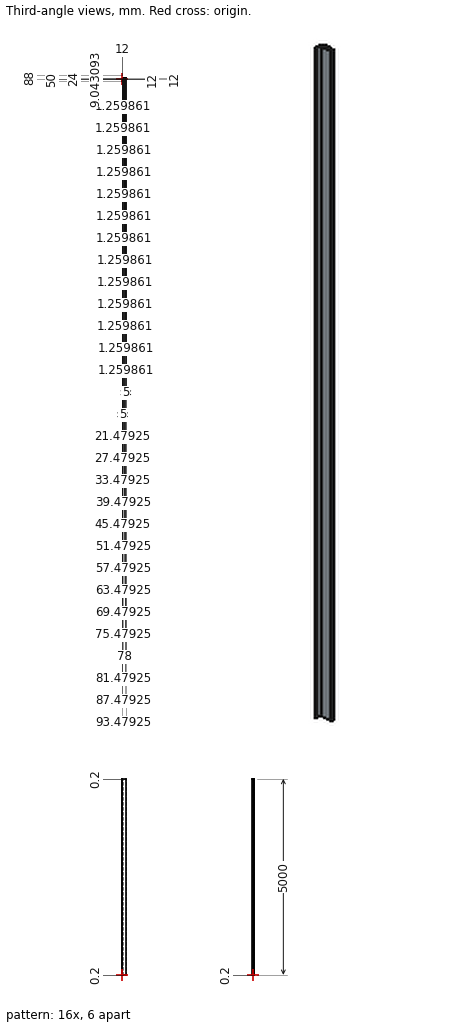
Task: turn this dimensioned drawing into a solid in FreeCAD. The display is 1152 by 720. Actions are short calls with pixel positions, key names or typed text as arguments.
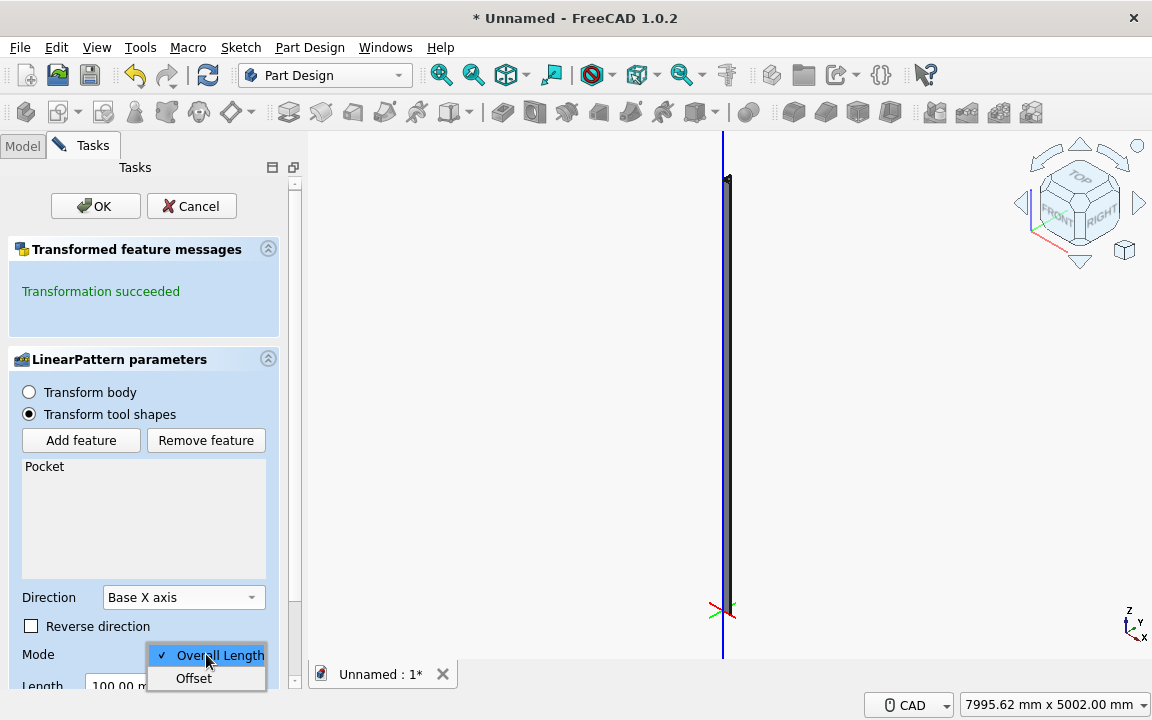
click(206, 678)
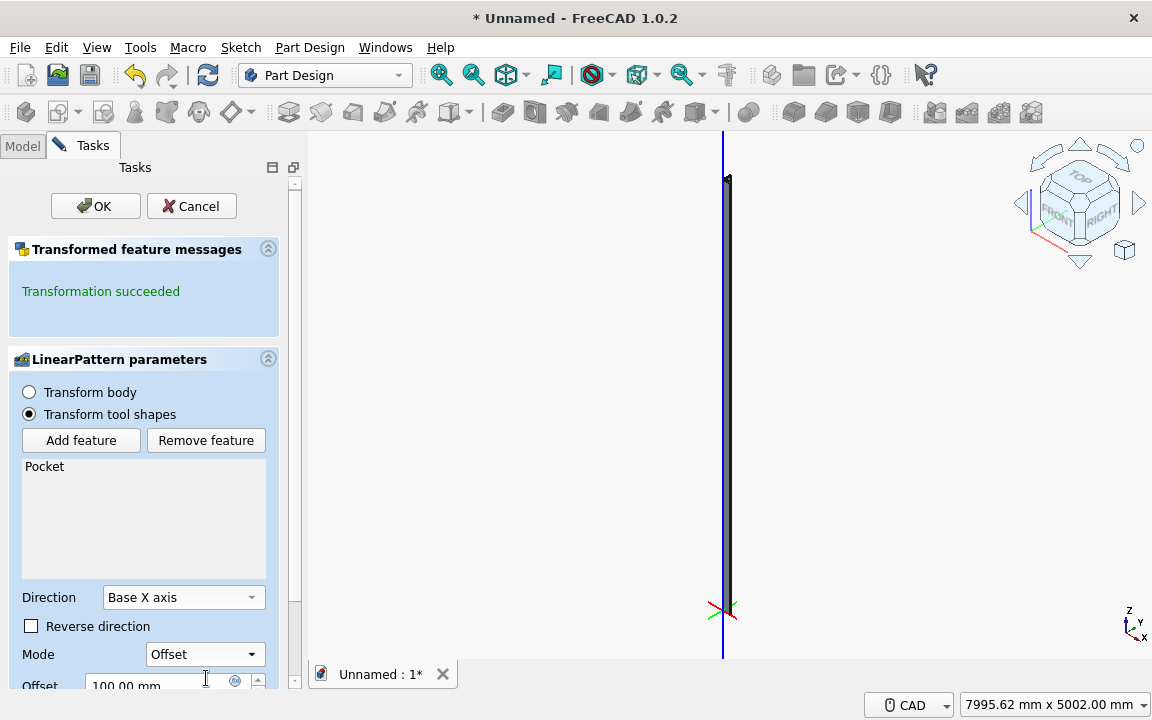
scroll(295, 432, down, 2)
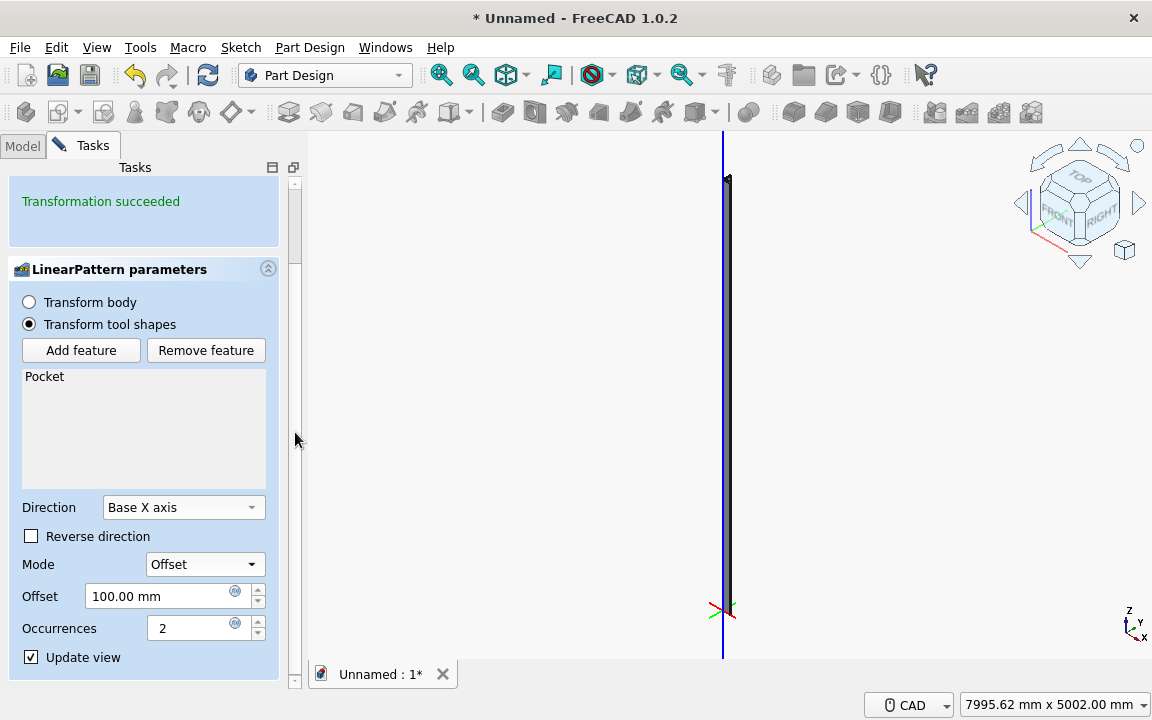
triple_click(168, 596)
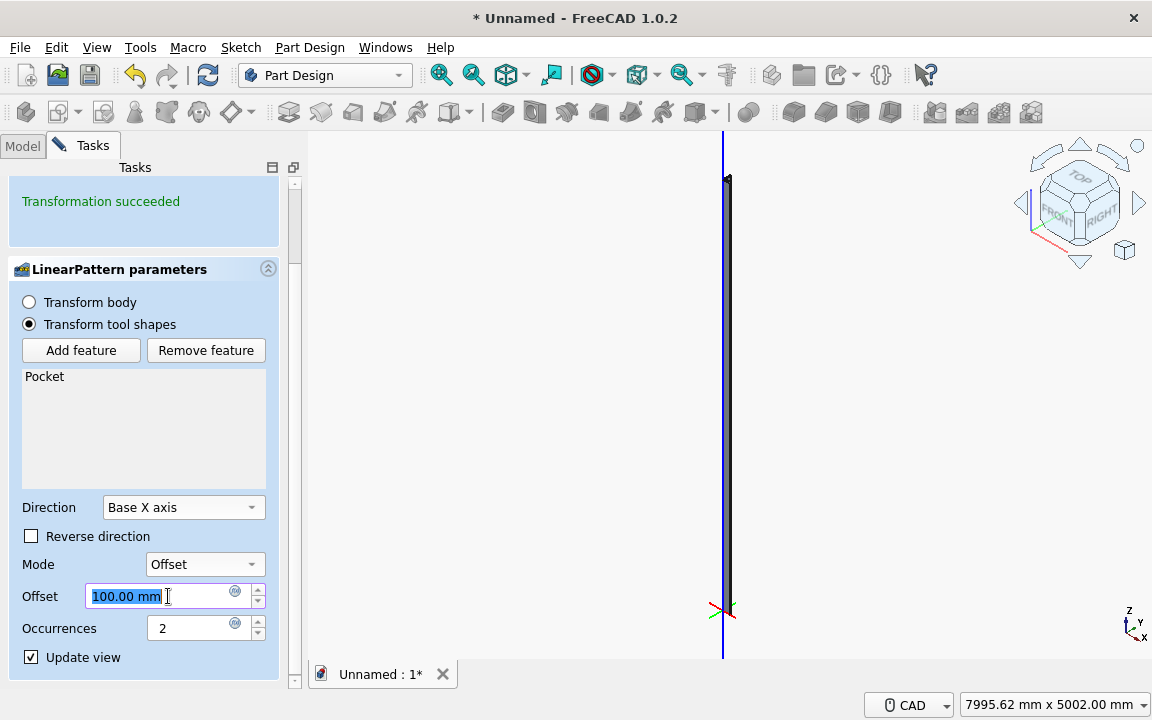
text(6)
key(Tab)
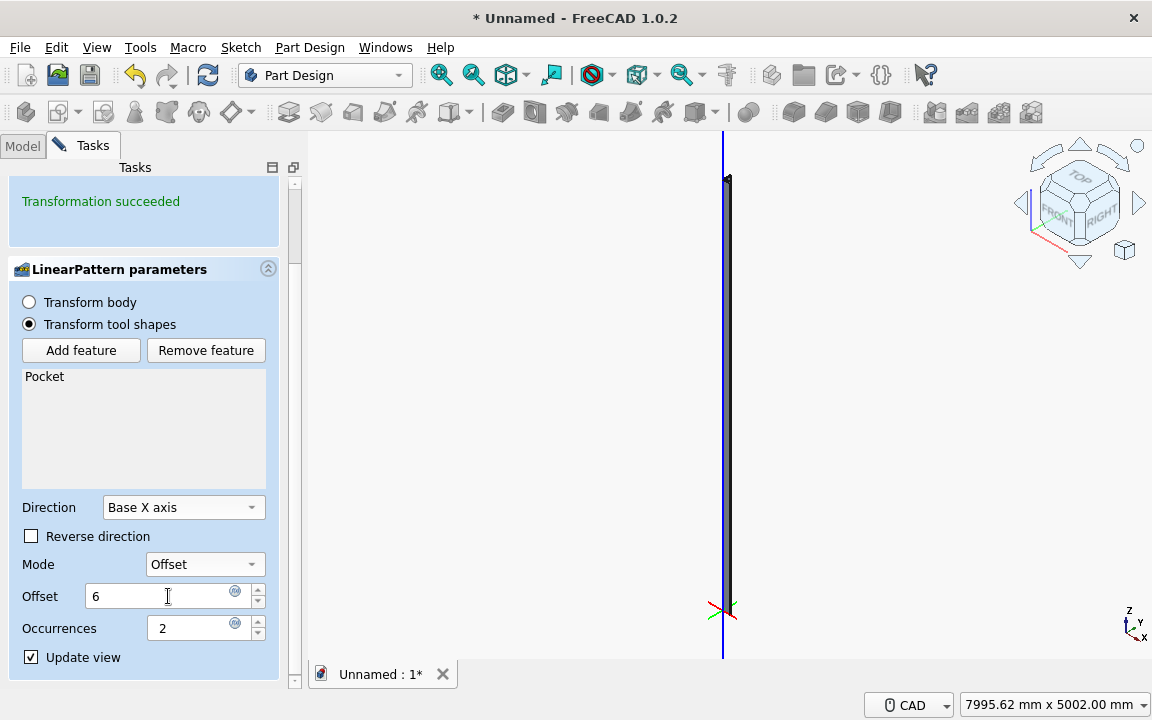
triple_click(198, 628)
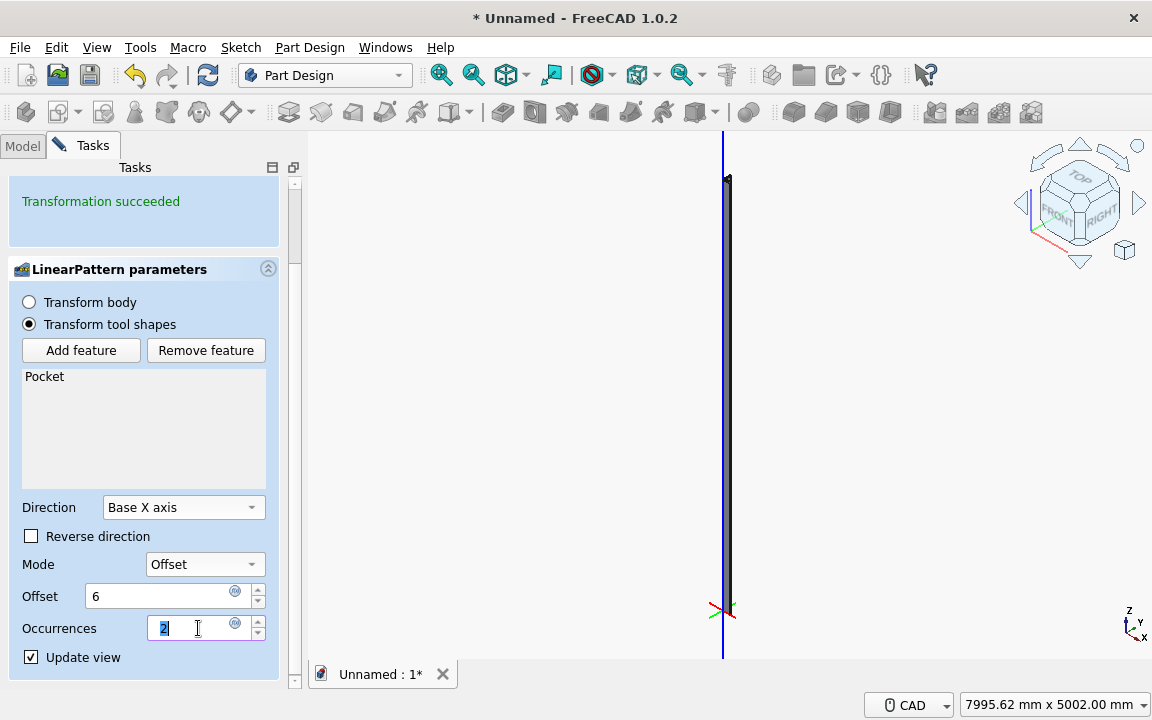
text(16)
key(Tab)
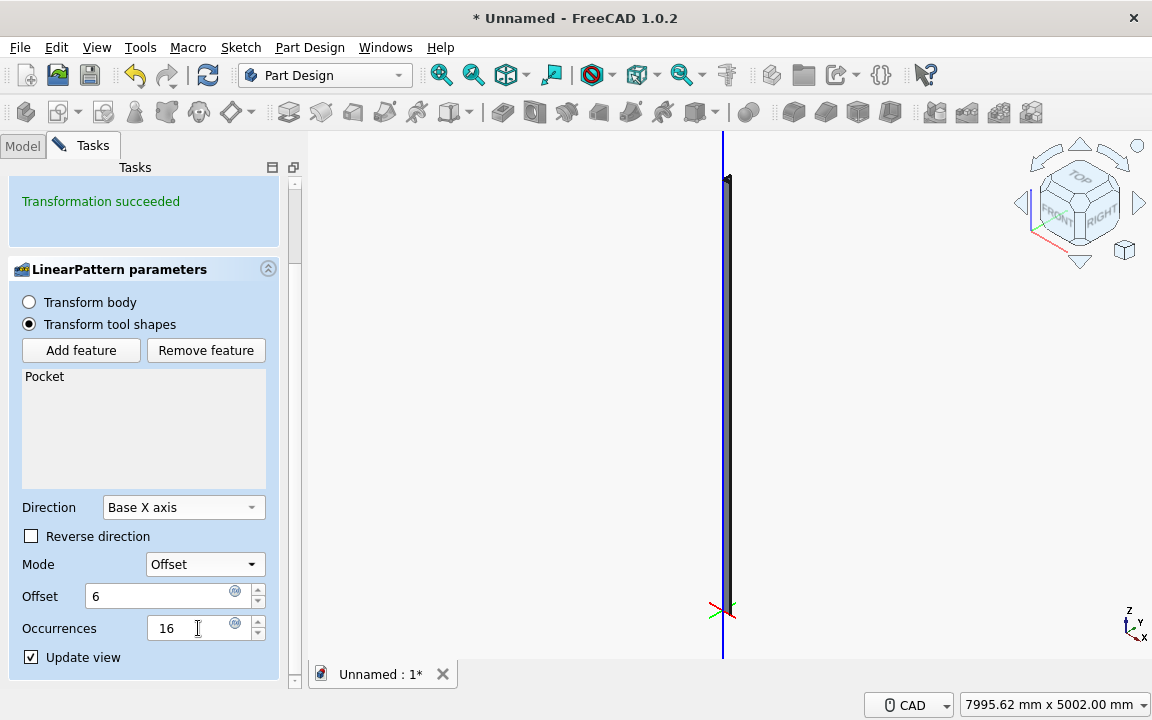
scroll(295, 432, up, 3)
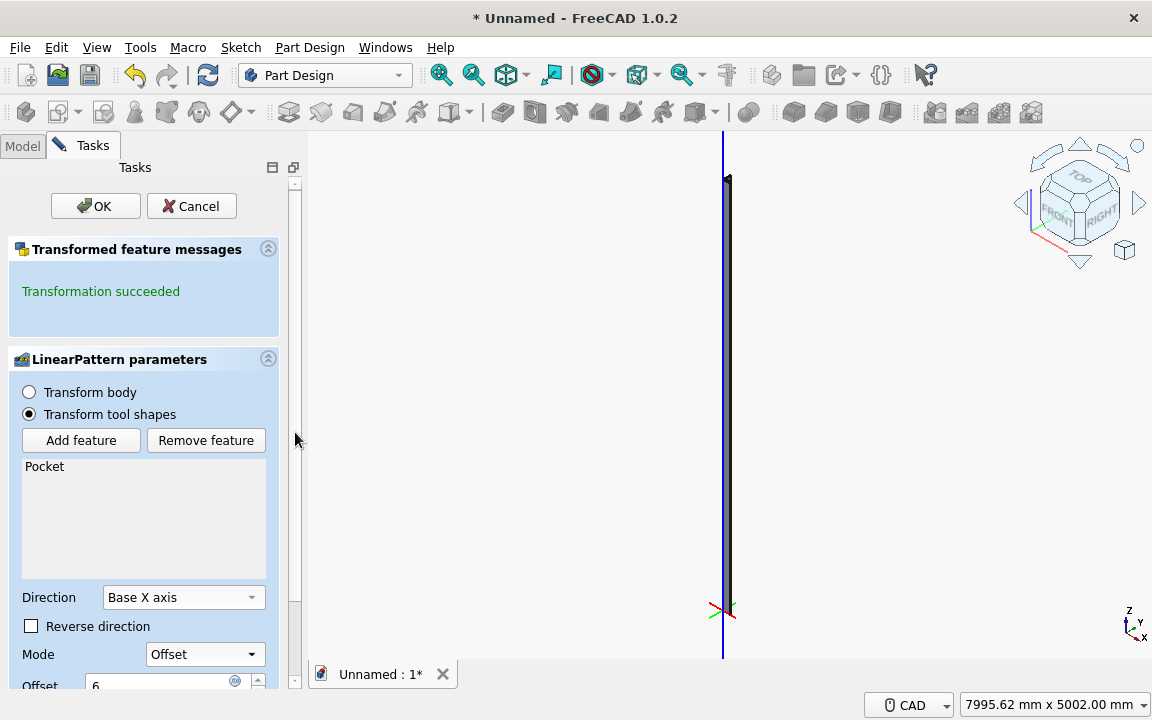
click(96, 206)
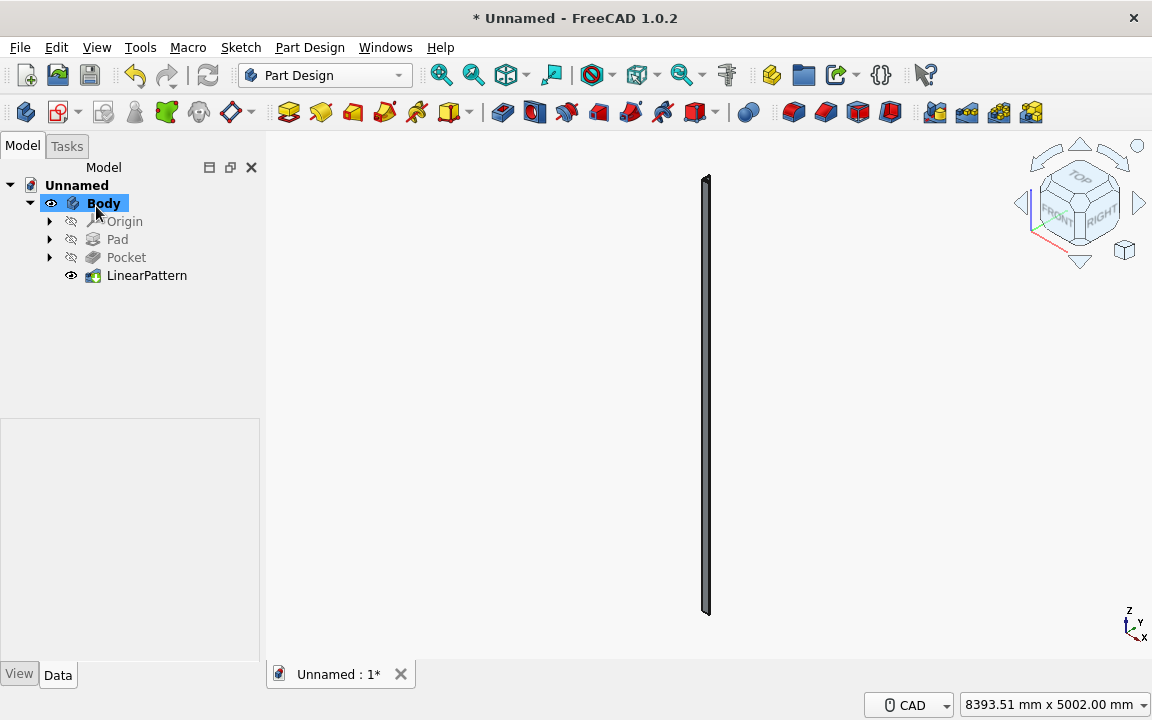
click(50, 221)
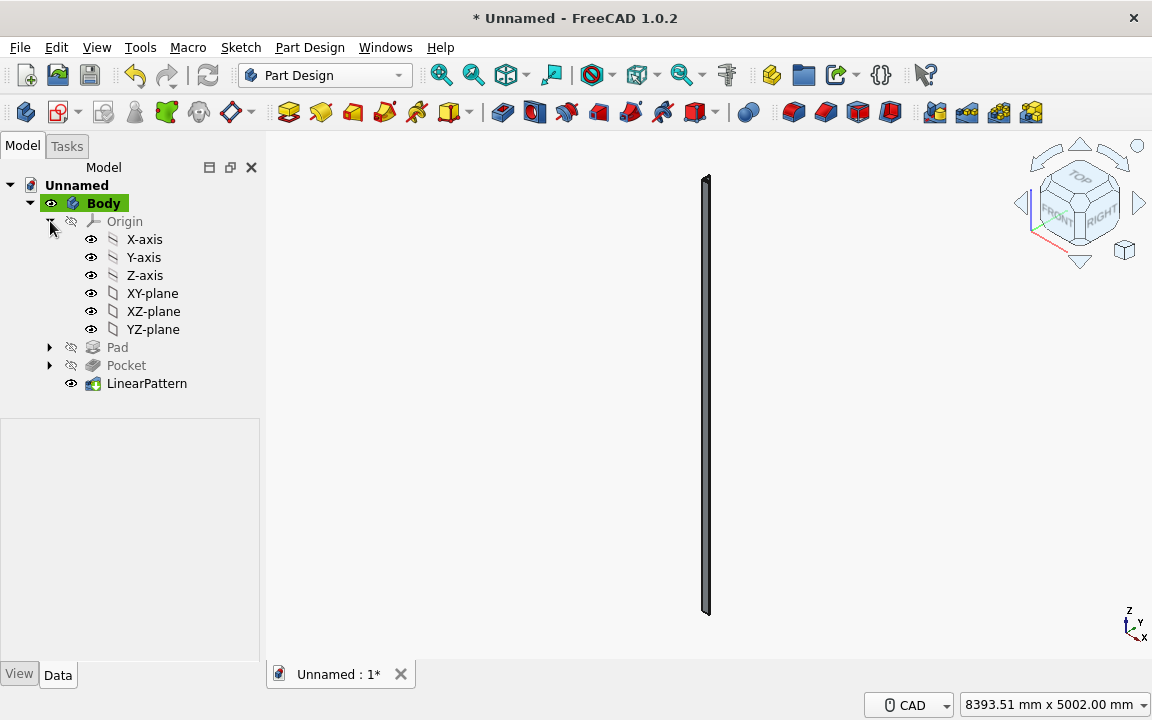
click(136, 293)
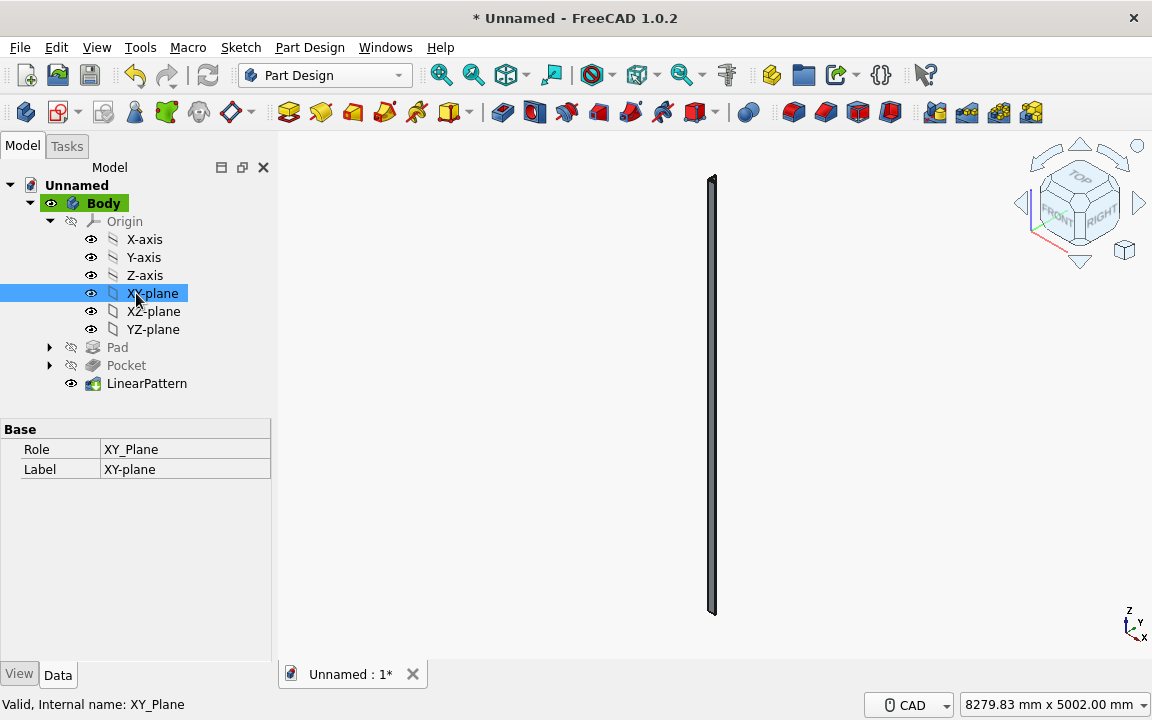
click(232, 112)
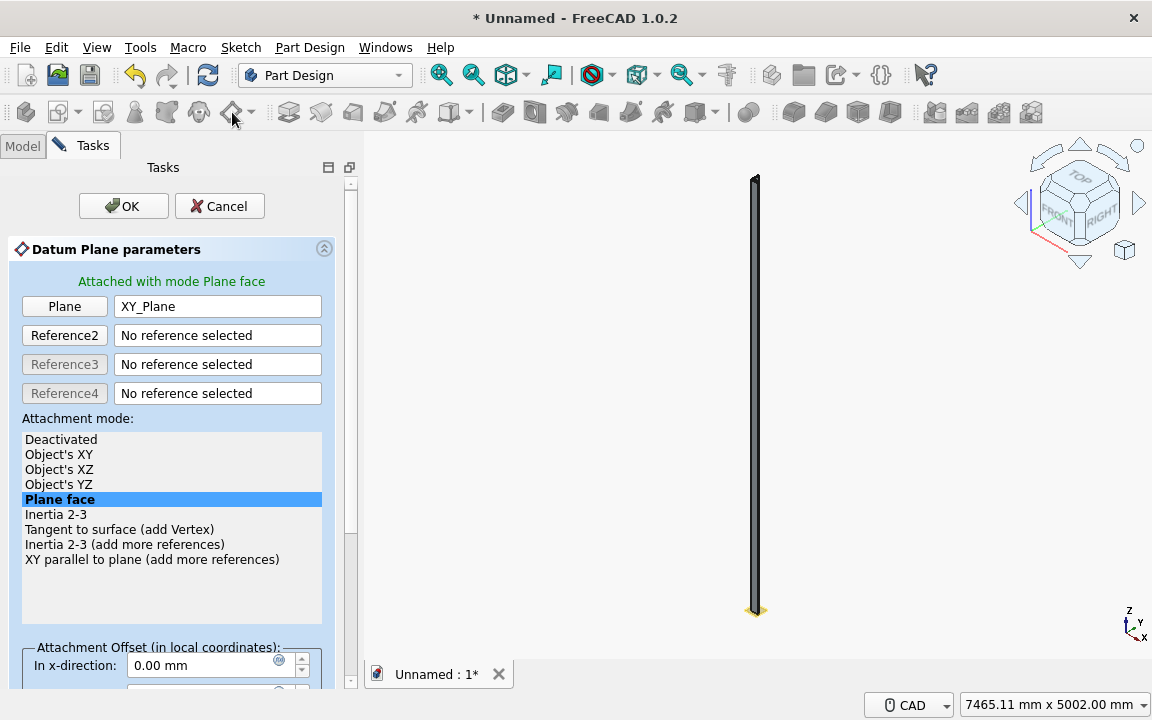
scroll(351, 432, down, 2)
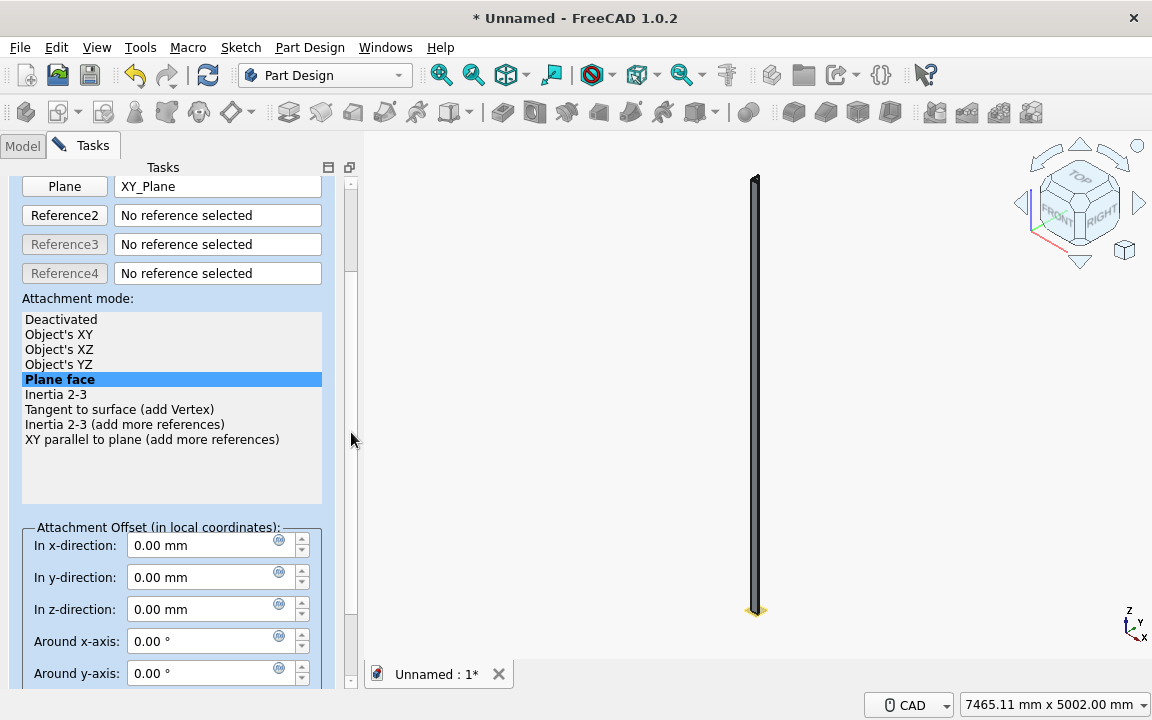
triple_click(210, 609)